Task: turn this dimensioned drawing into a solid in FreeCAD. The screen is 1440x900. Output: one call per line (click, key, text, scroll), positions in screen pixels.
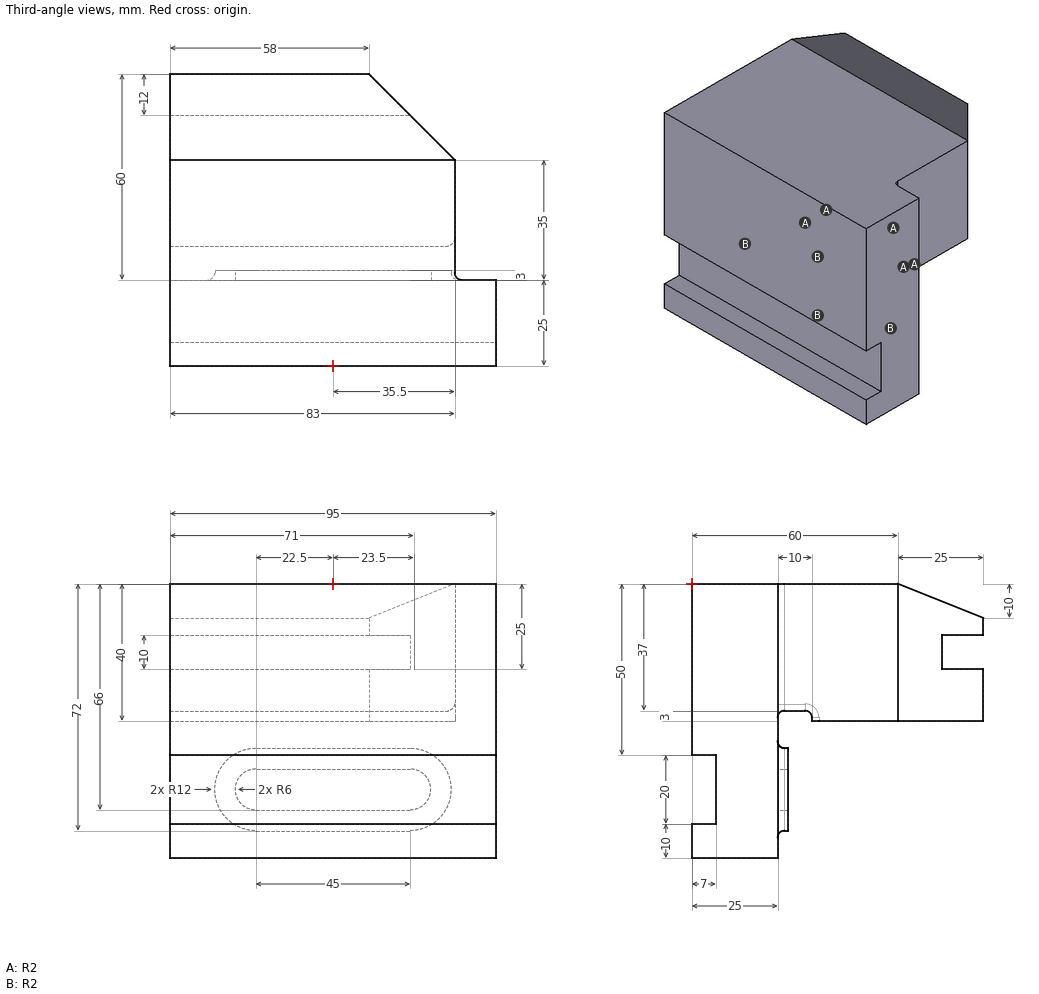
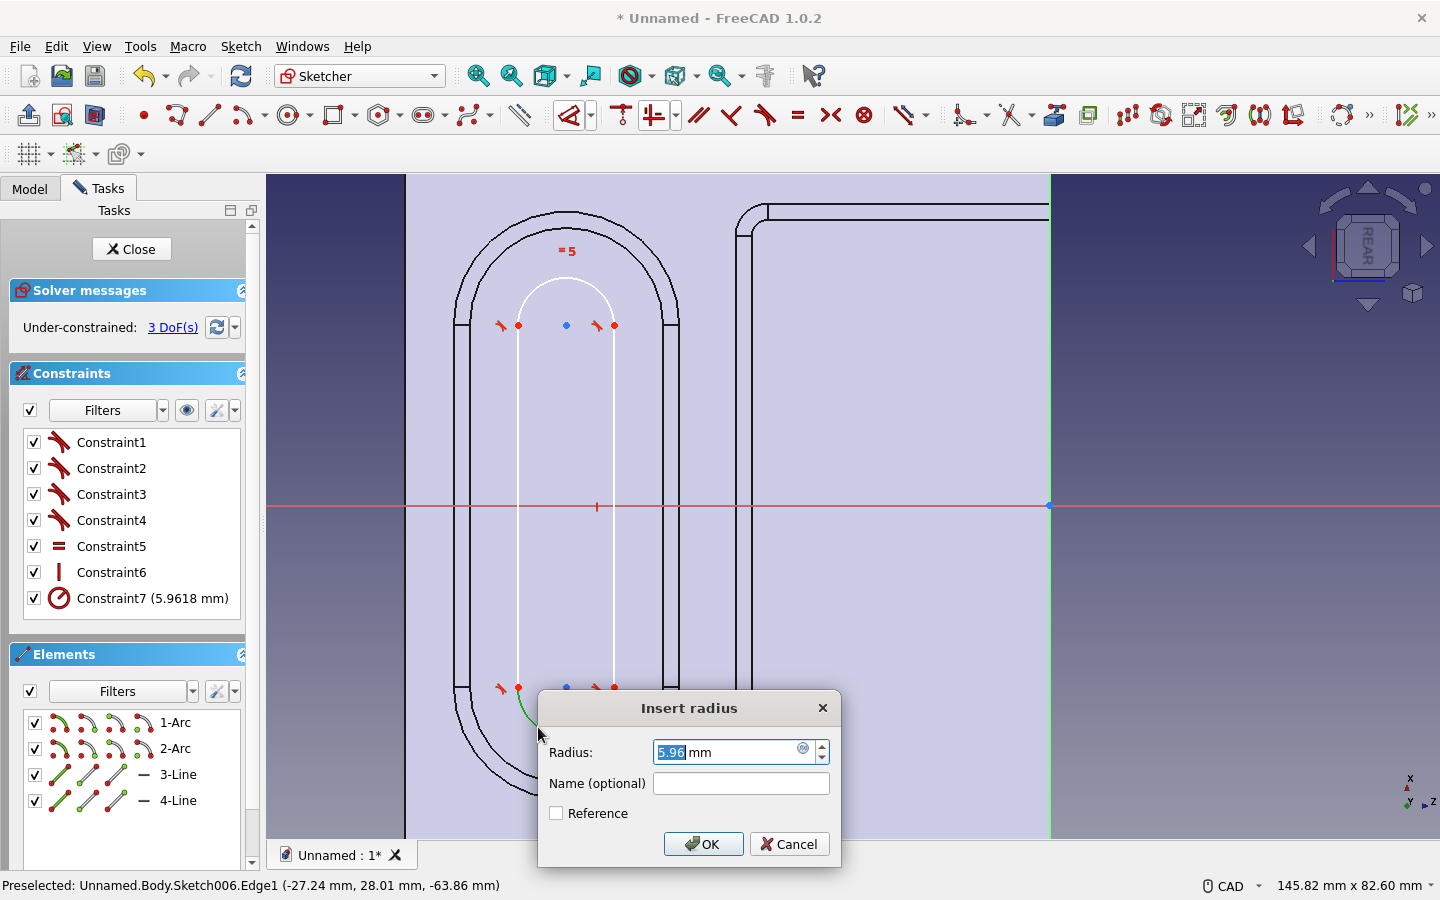
text(6)
key(Return)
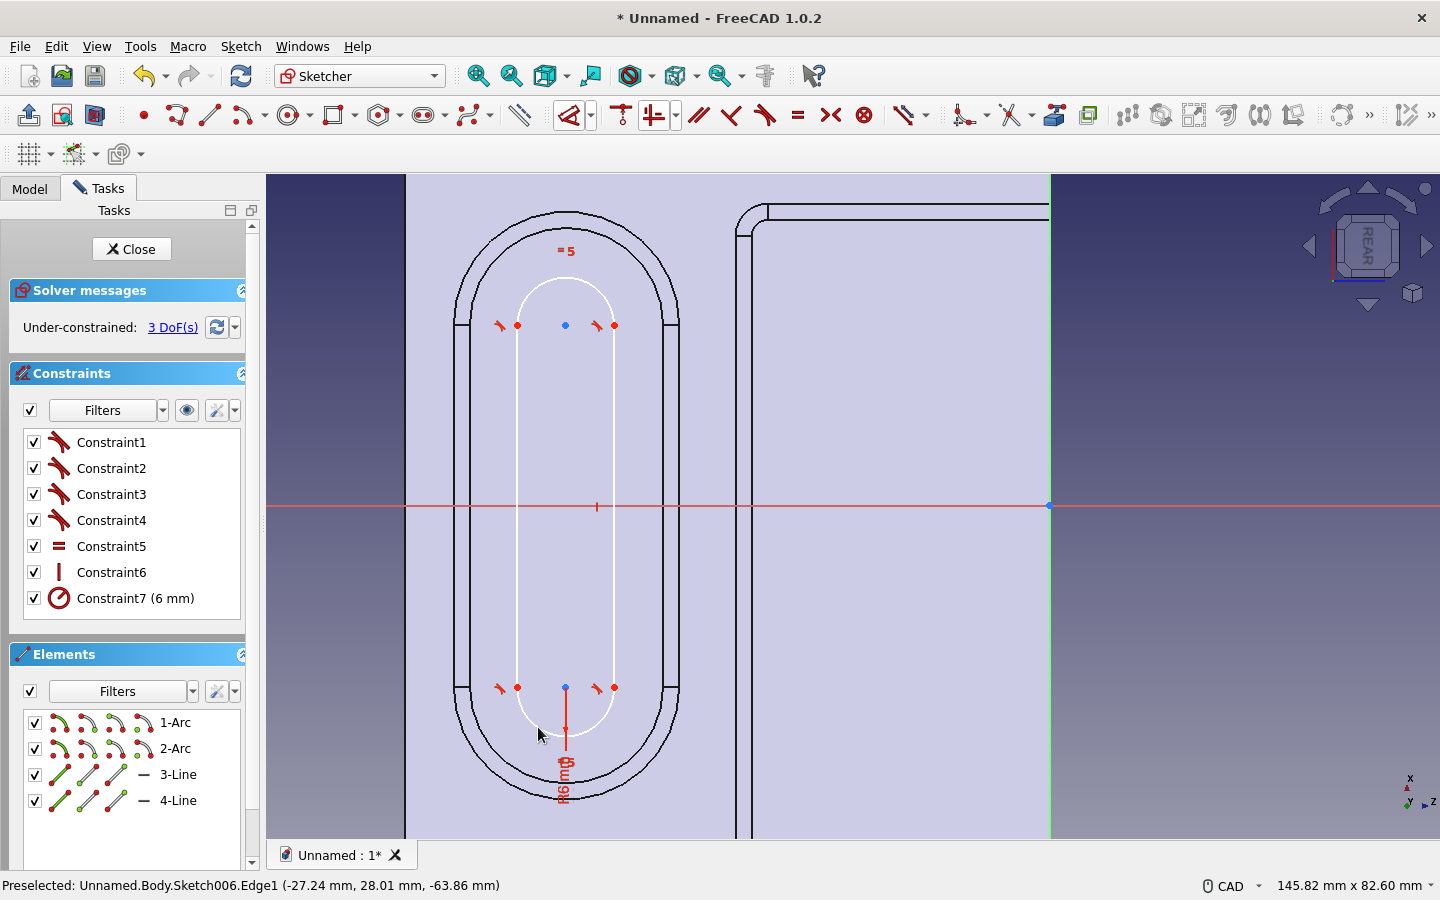
click(517, 579)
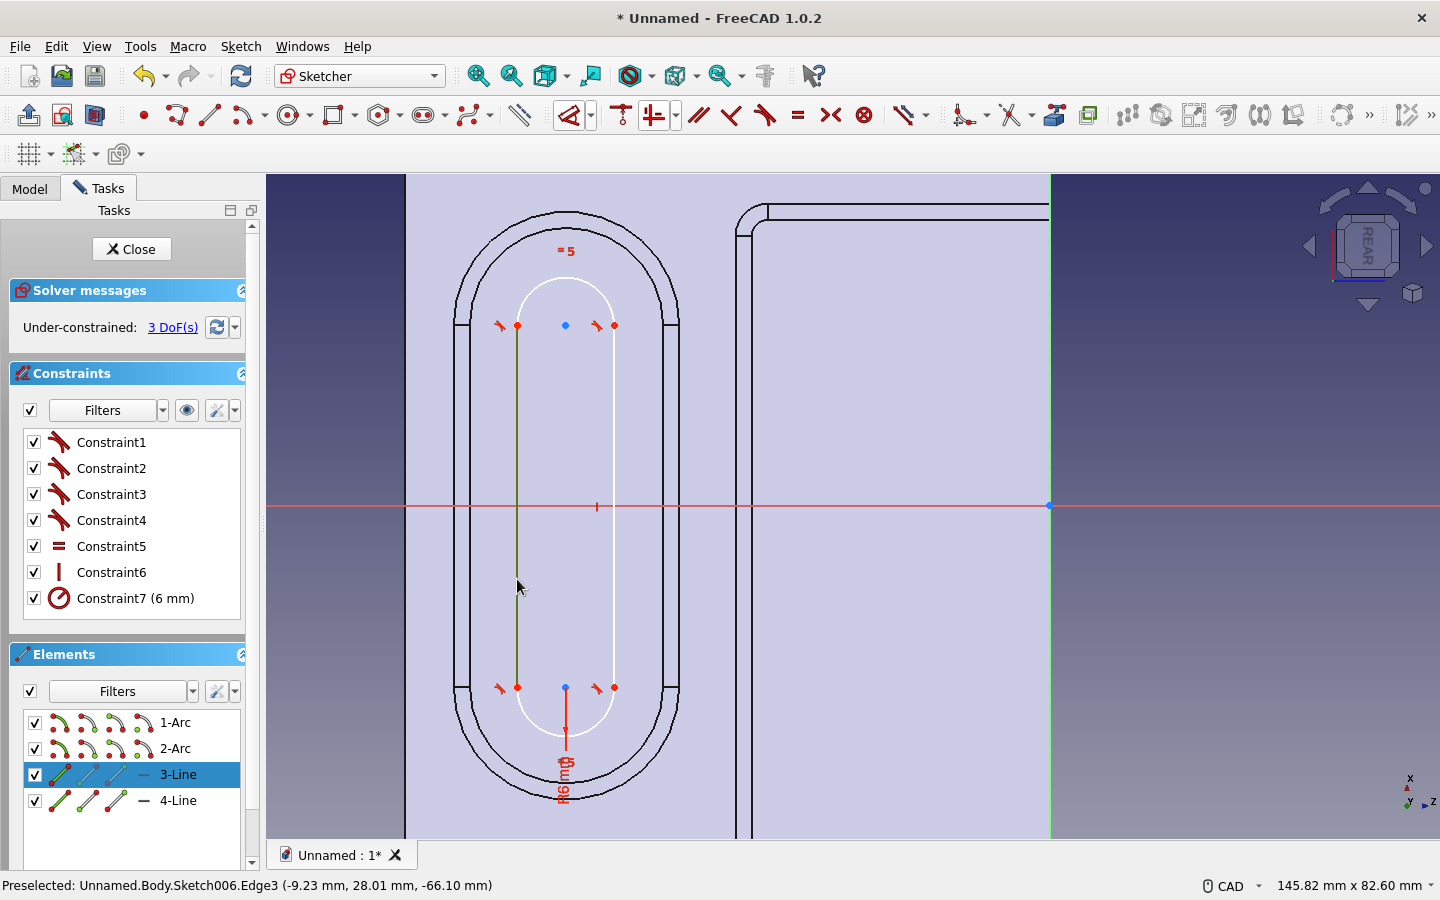
click(590, 116)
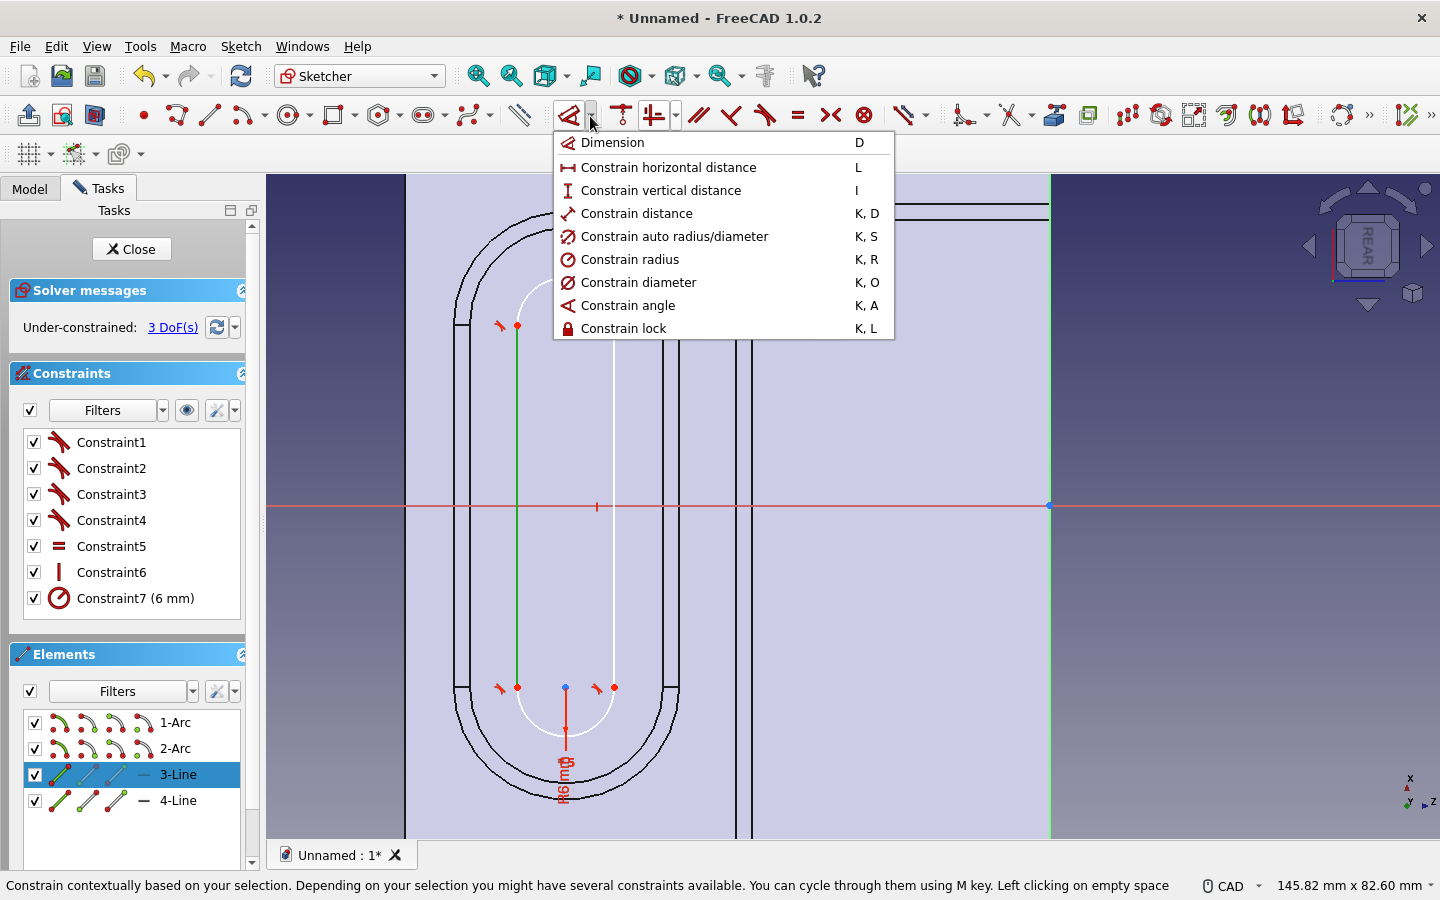
click(724, 190)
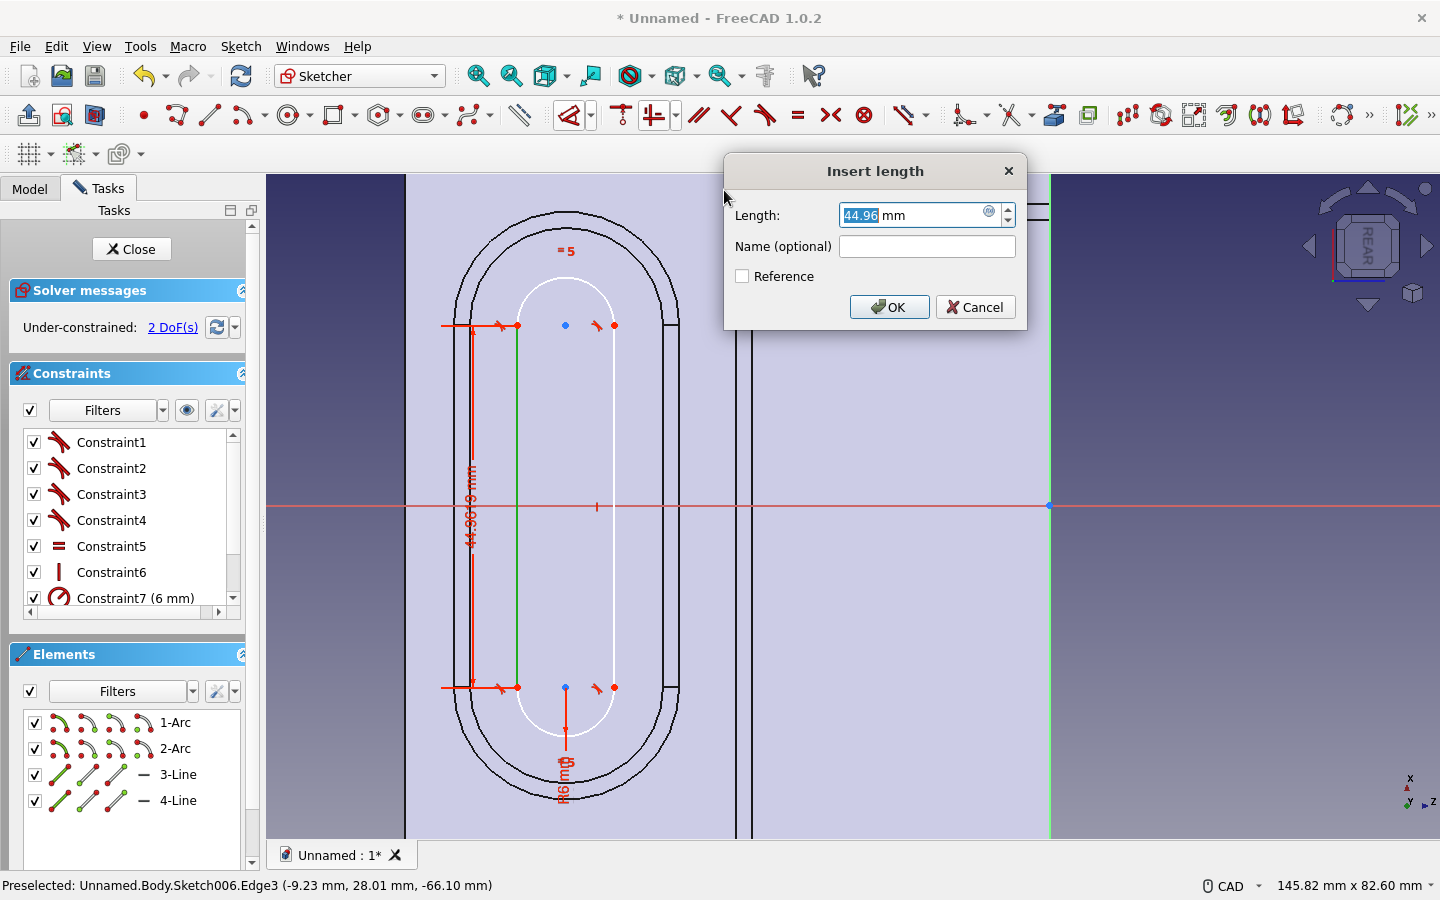
text(45)
key(Return)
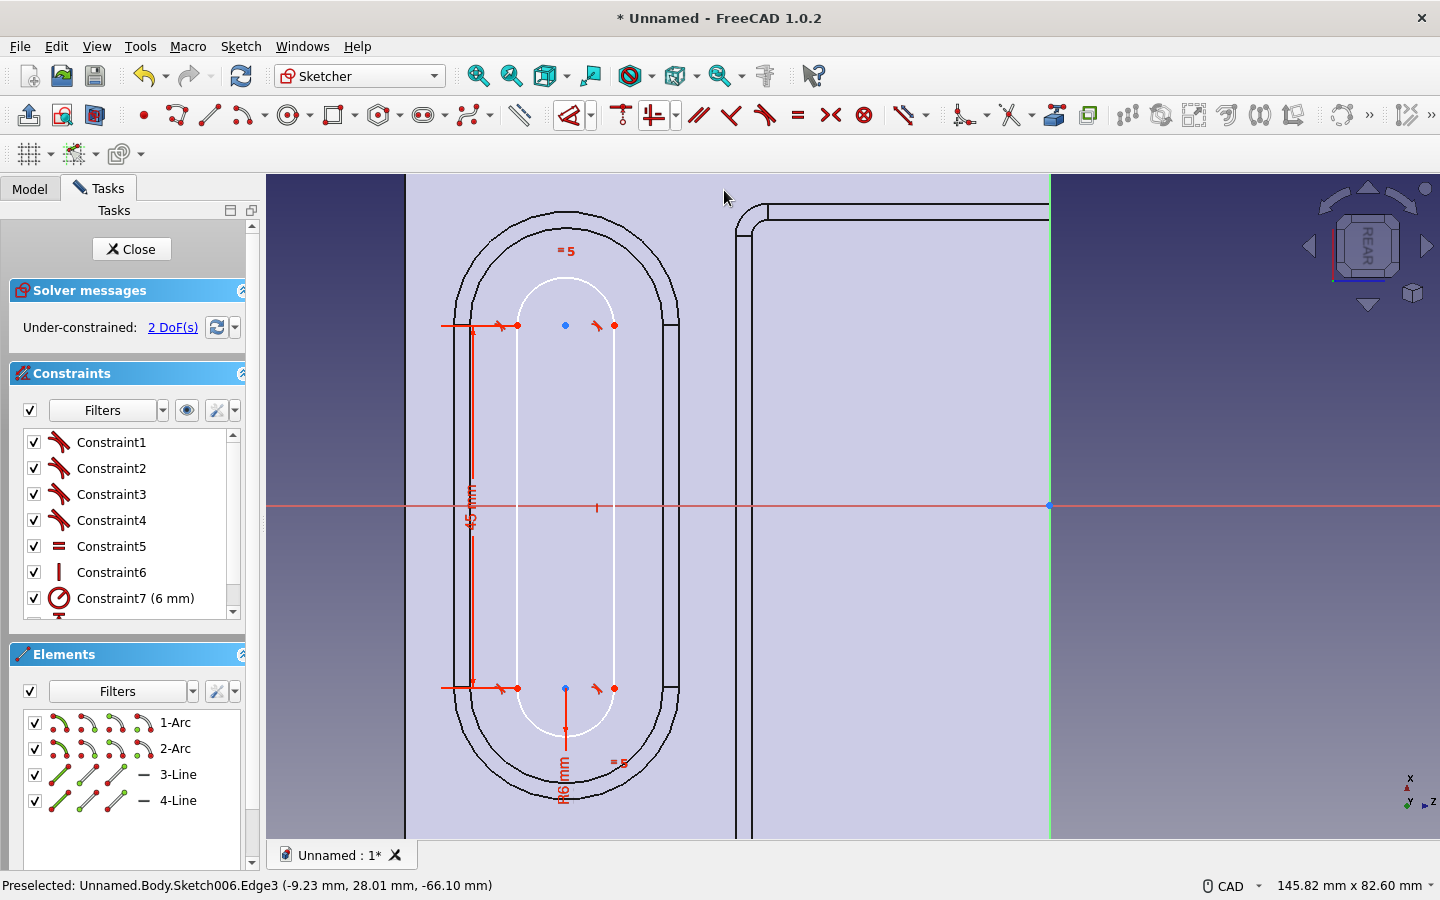
click(517, 688)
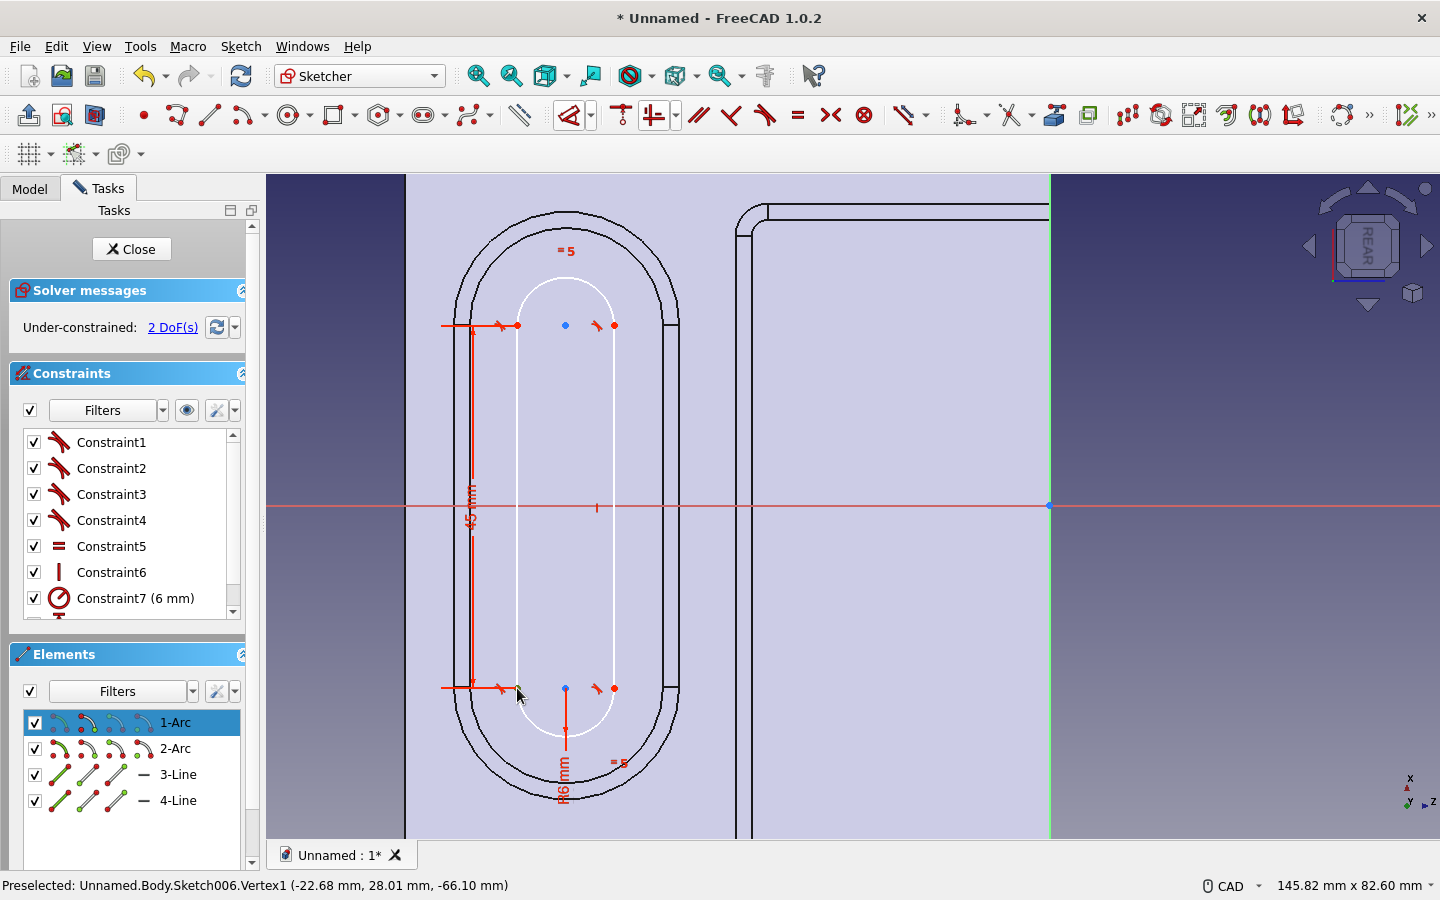
key(l)